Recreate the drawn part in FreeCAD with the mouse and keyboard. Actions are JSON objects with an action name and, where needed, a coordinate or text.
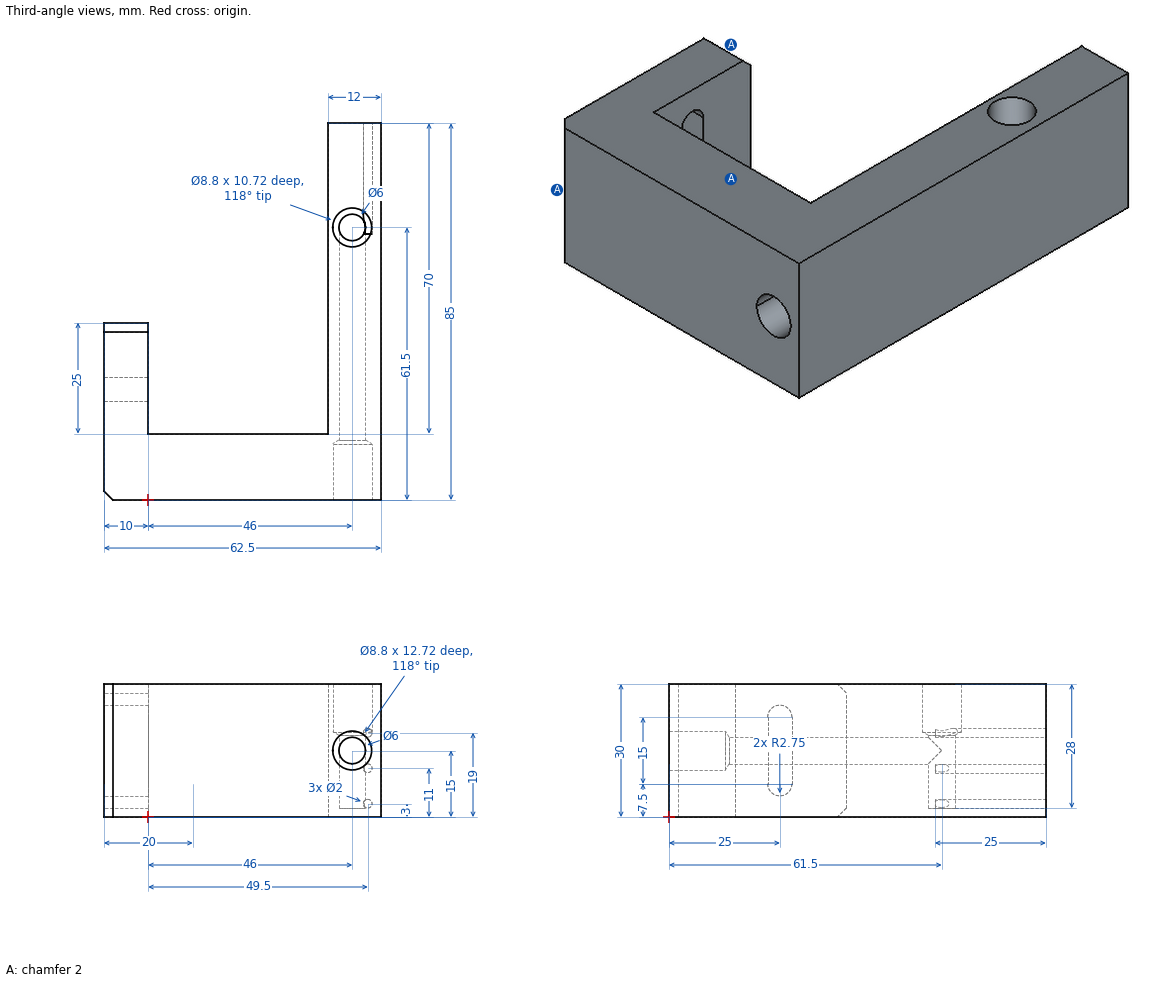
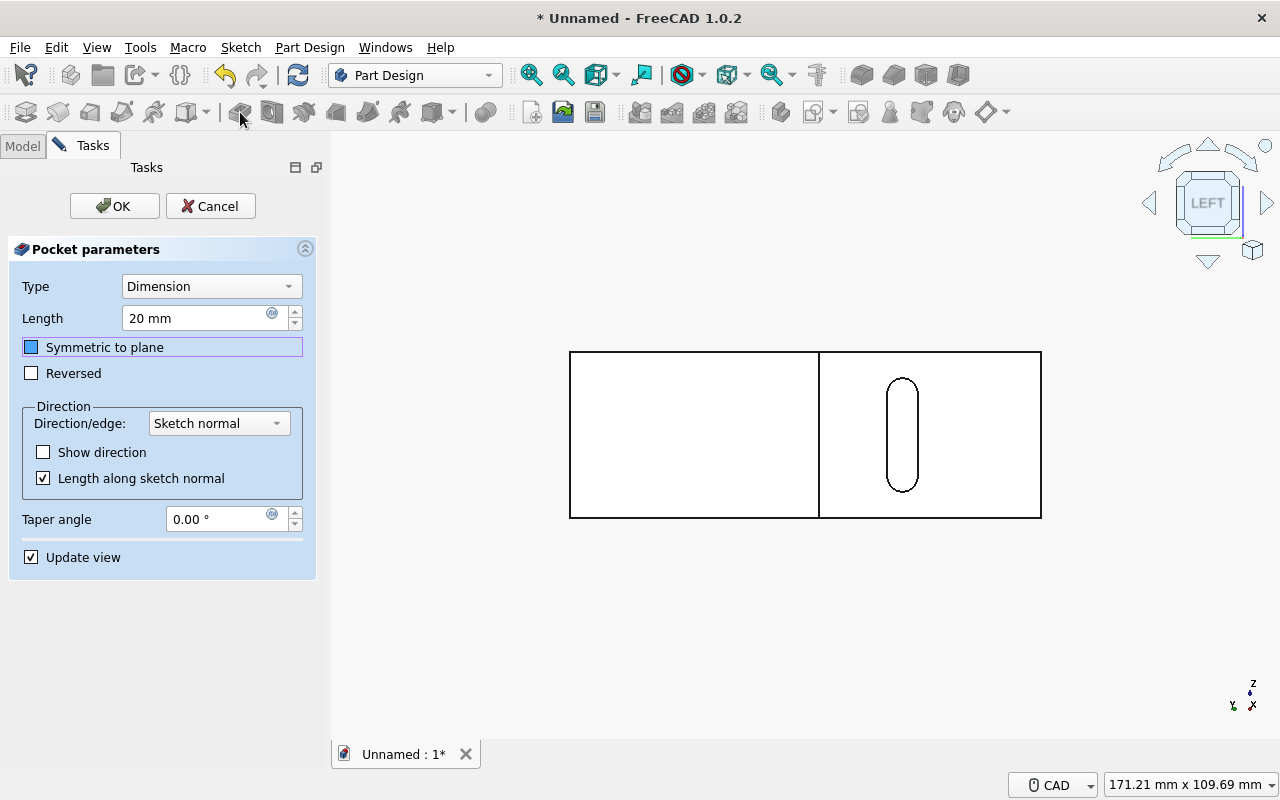
{"action": "left_click", "coordinate": [115, 206]}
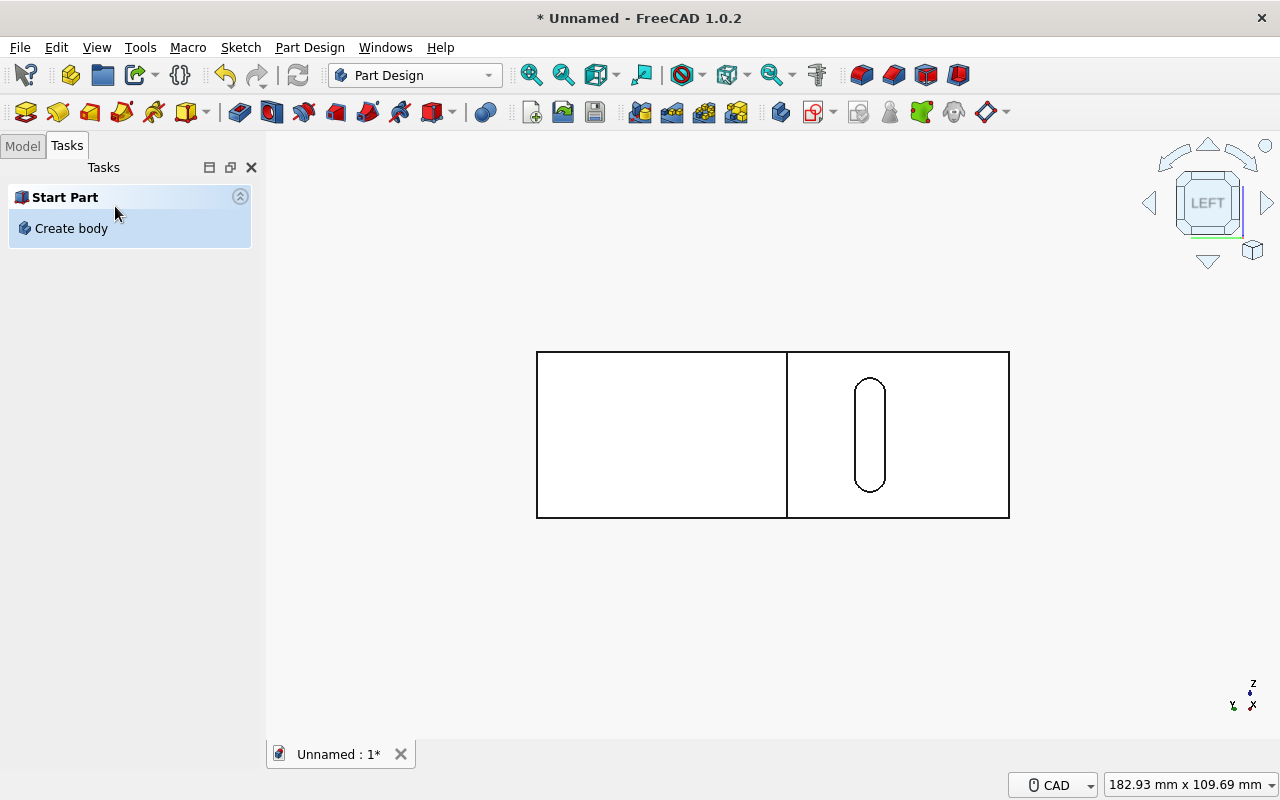
{"action": "left_click", "coordinate": [1009, 434]}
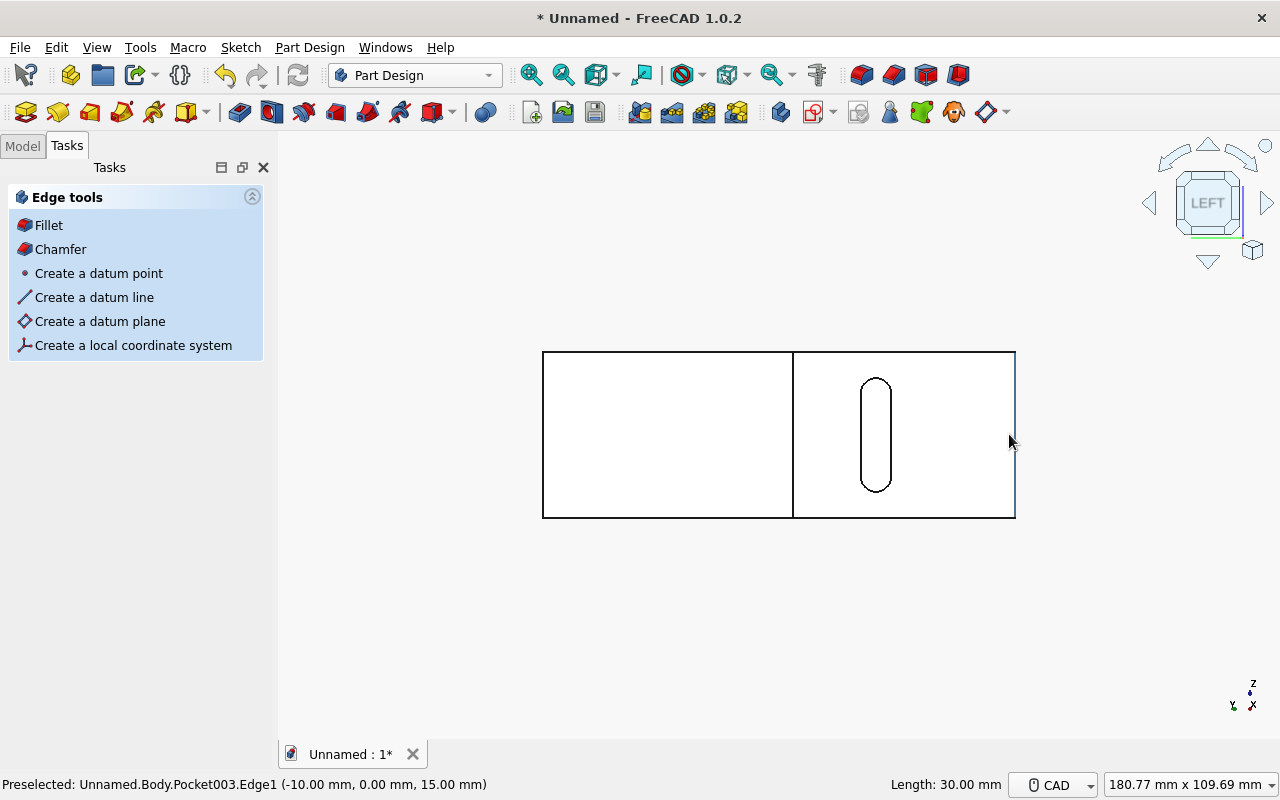
{"action": "key", "text": "0"}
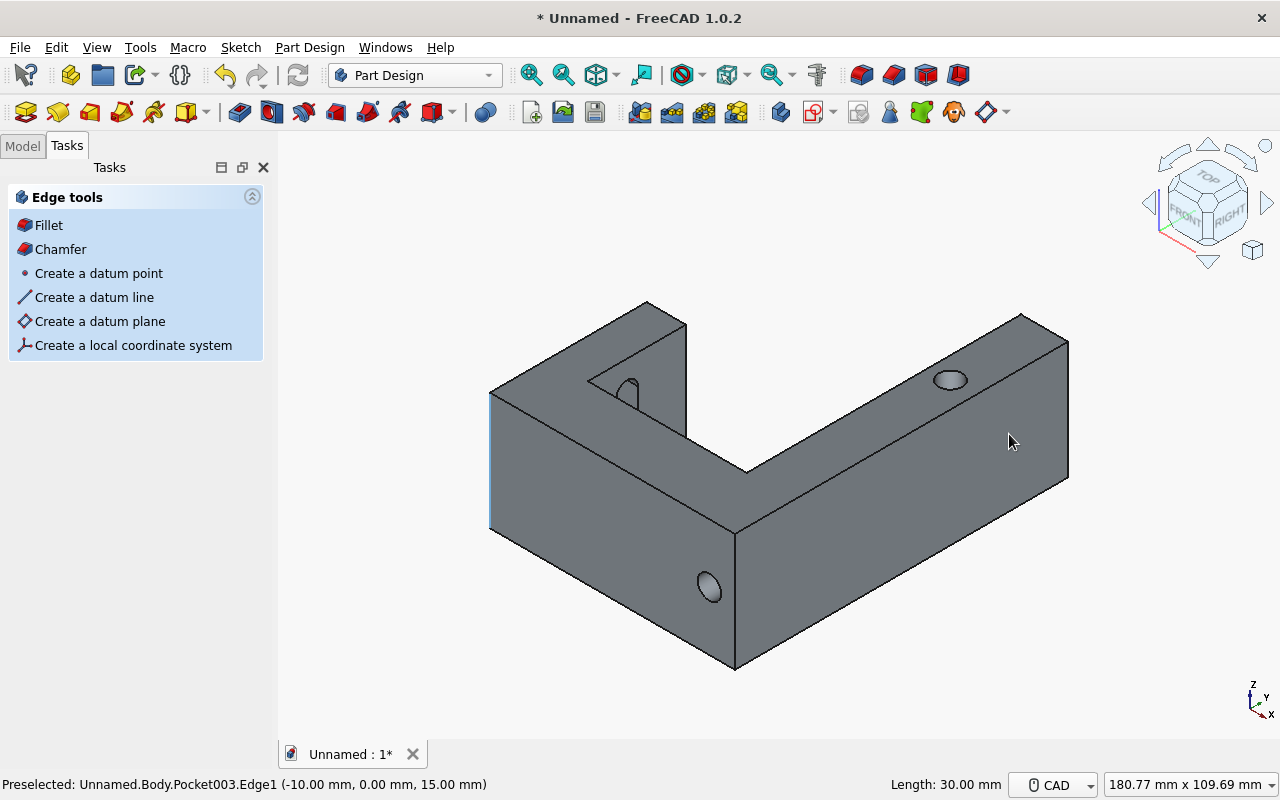
{"action": "key", "text": "2"}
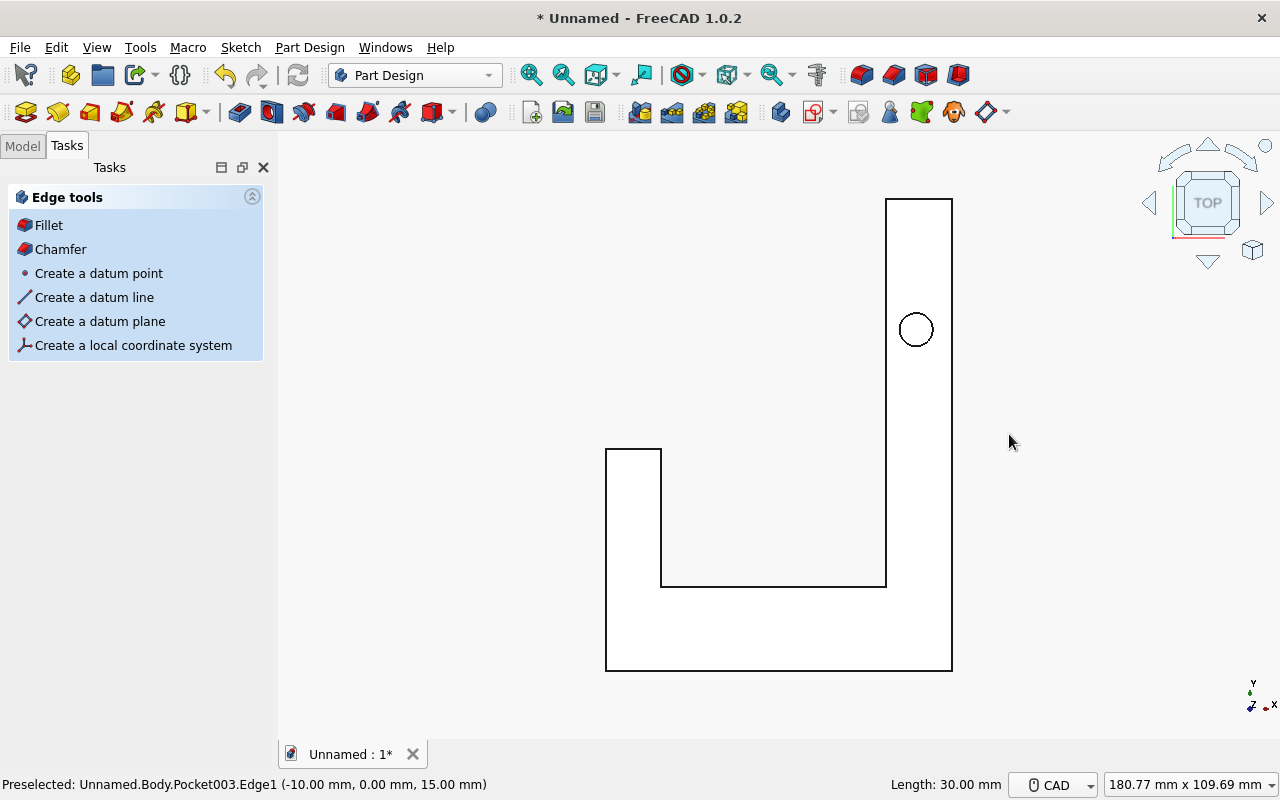
{"action": "left_click", "coordinate": [633, 448], "text": "ctrl"}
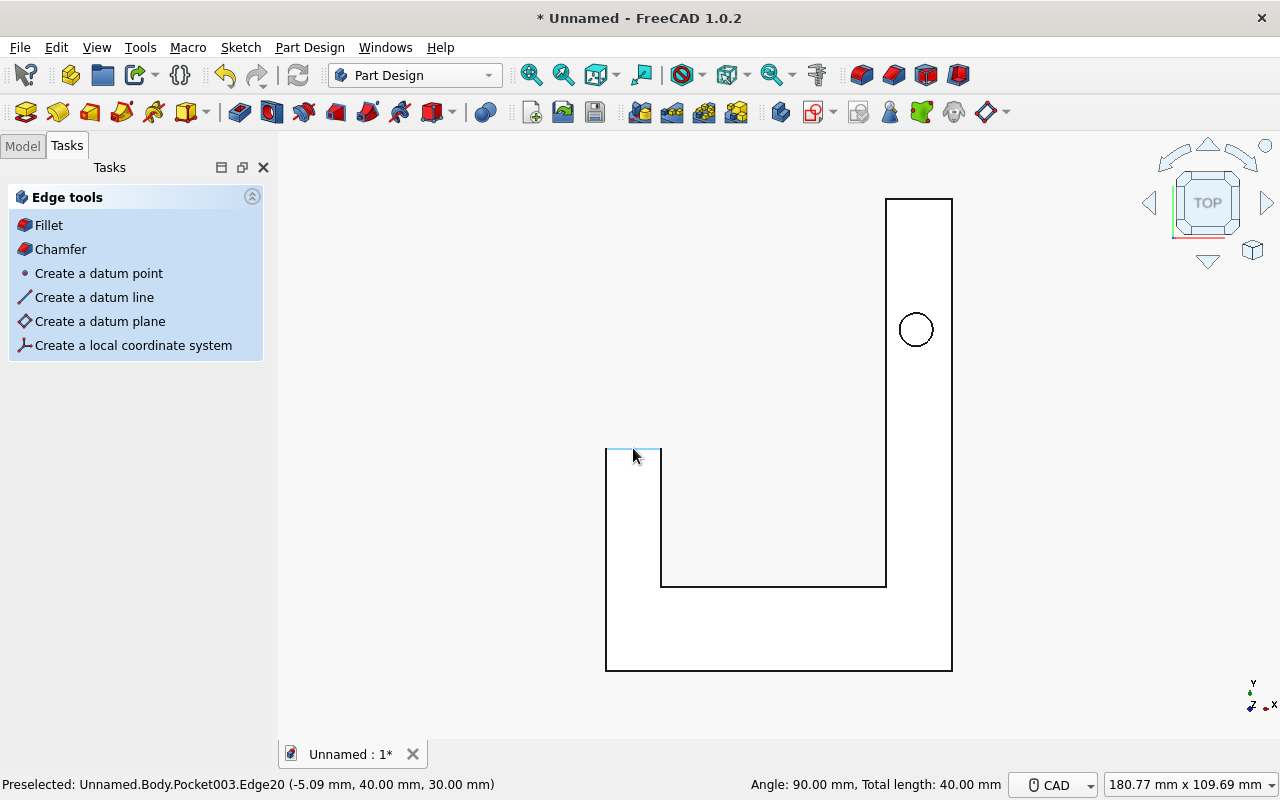
{"action": "key", "text": "1"}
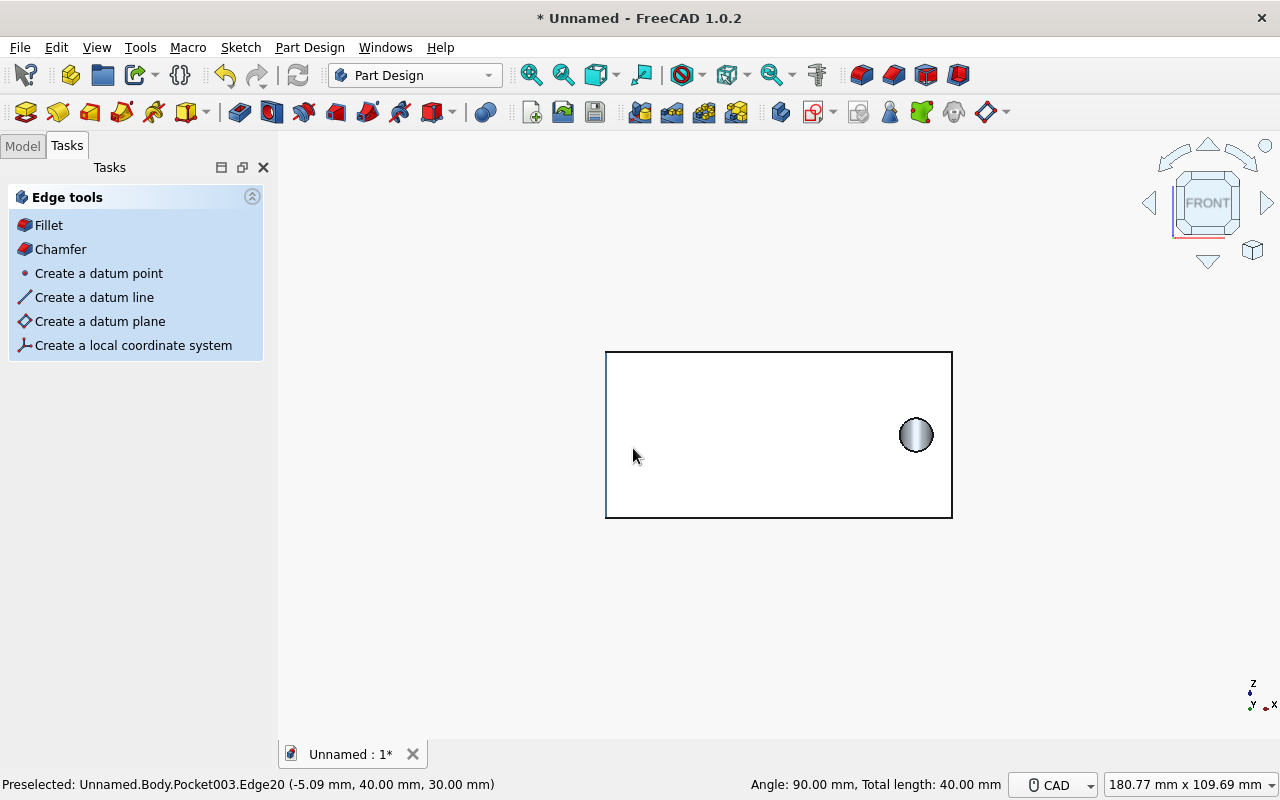
{"action": "key", "text": "v f"}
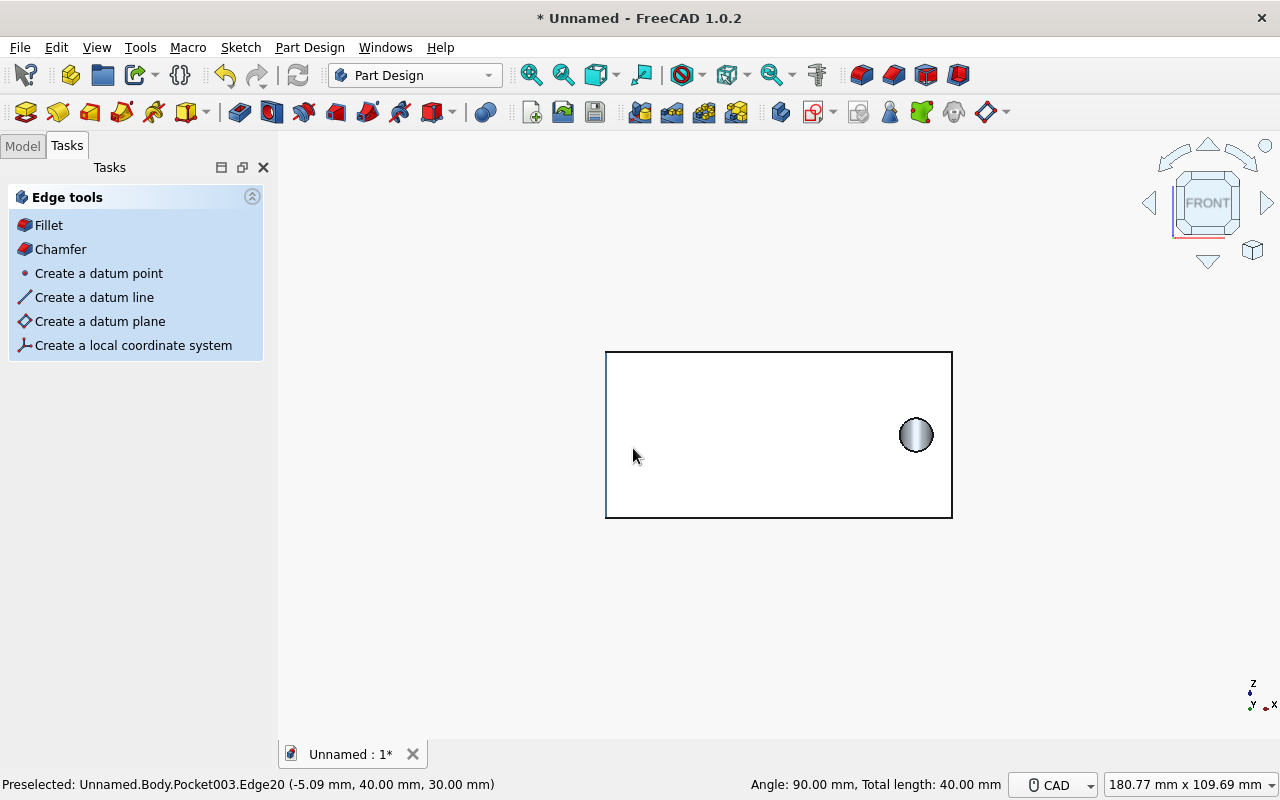
{"action": "key", "text": "3"}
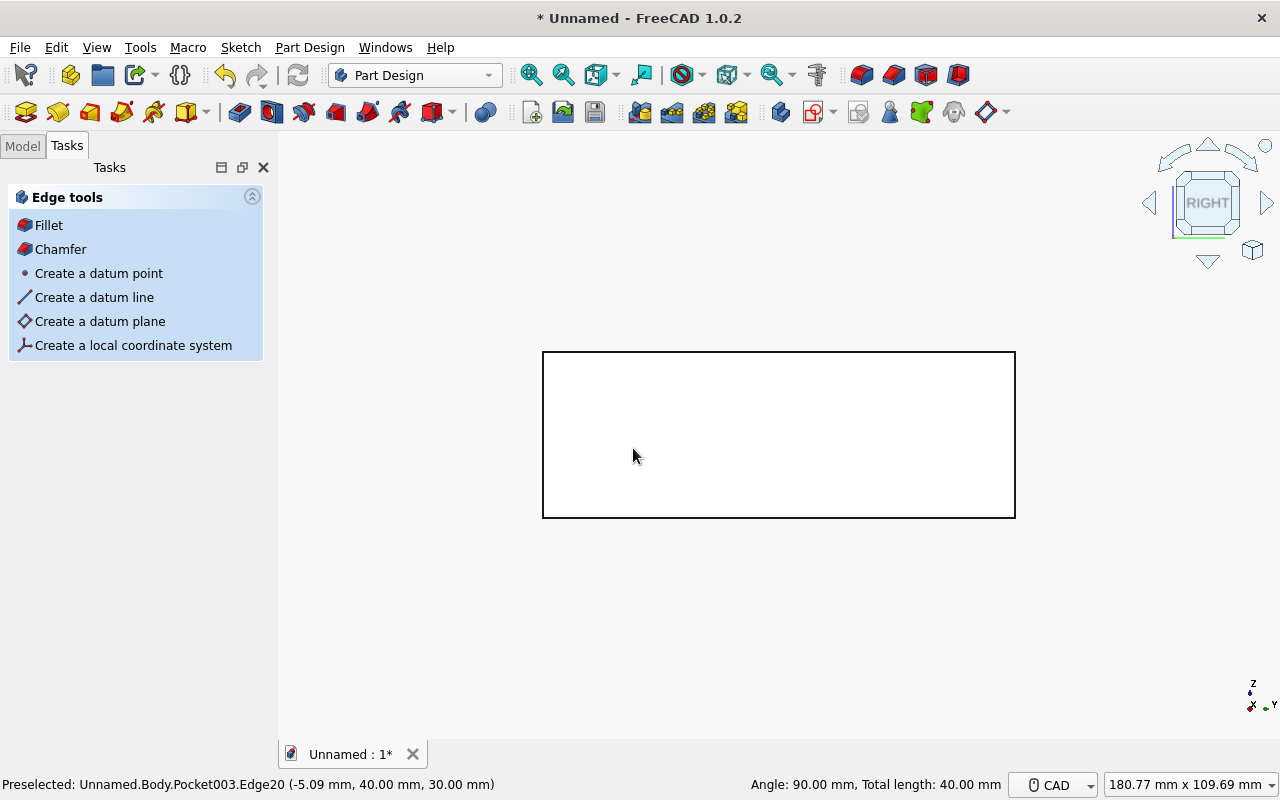
{"action": "key", "text": "5"}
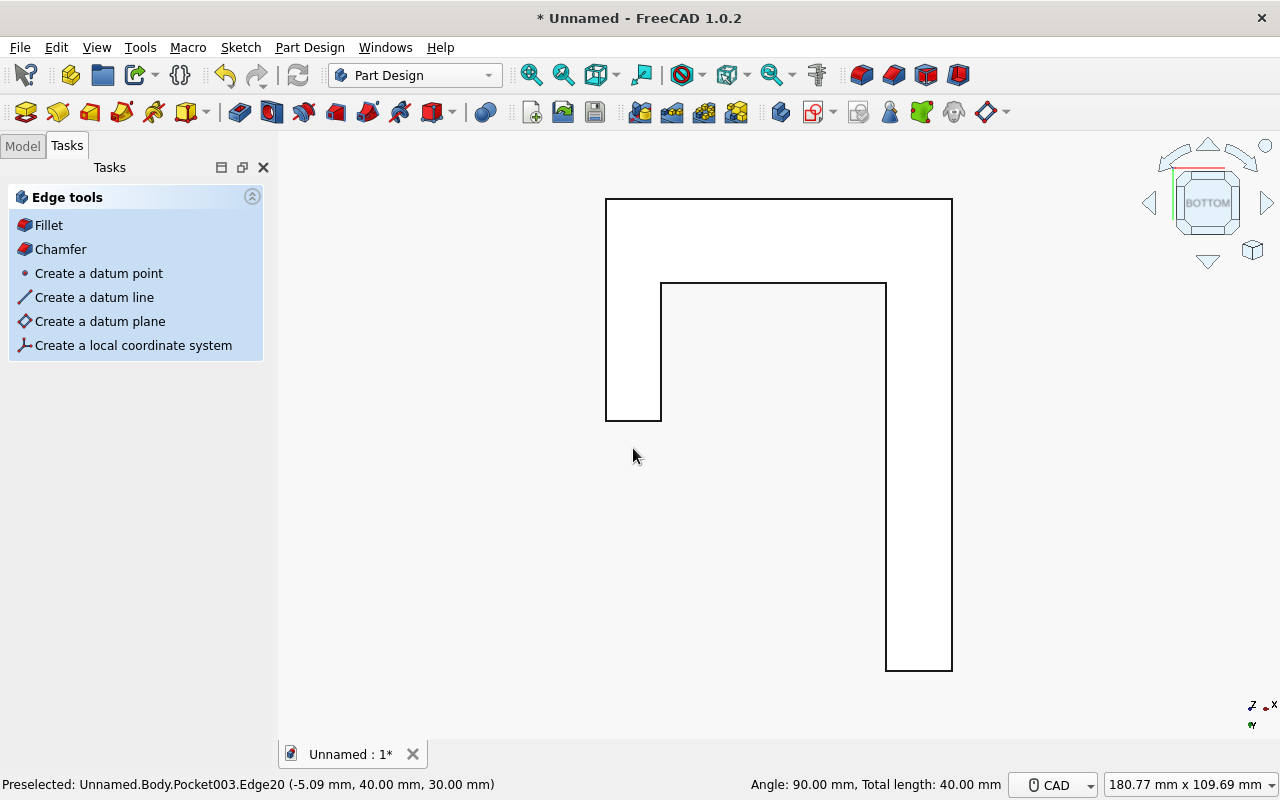
{"action": "left_click", "coordinate": [633, 420], "text": "ctrl"}